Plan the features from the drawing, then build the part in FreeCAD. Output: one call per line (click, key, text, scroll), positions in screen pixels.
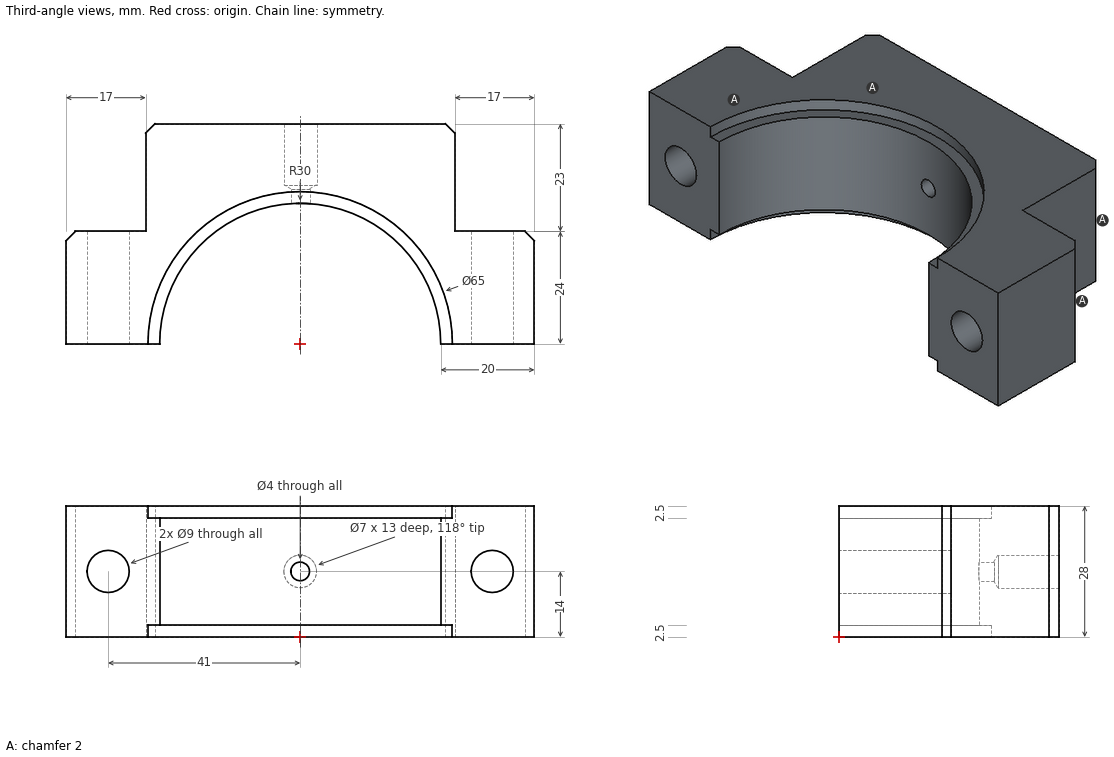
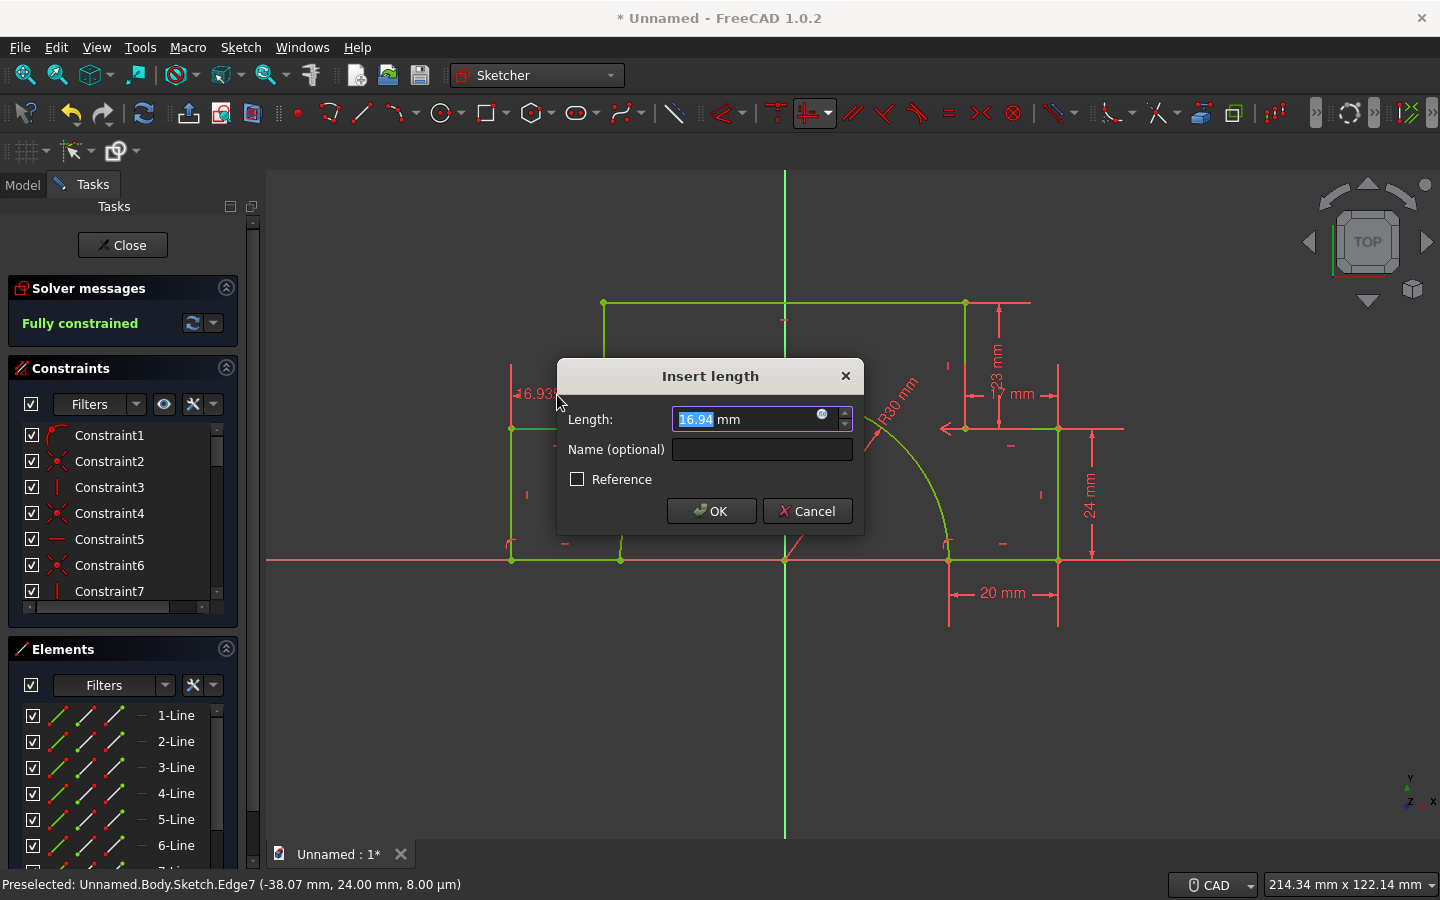
text(17)
key(Return)
key(Escape)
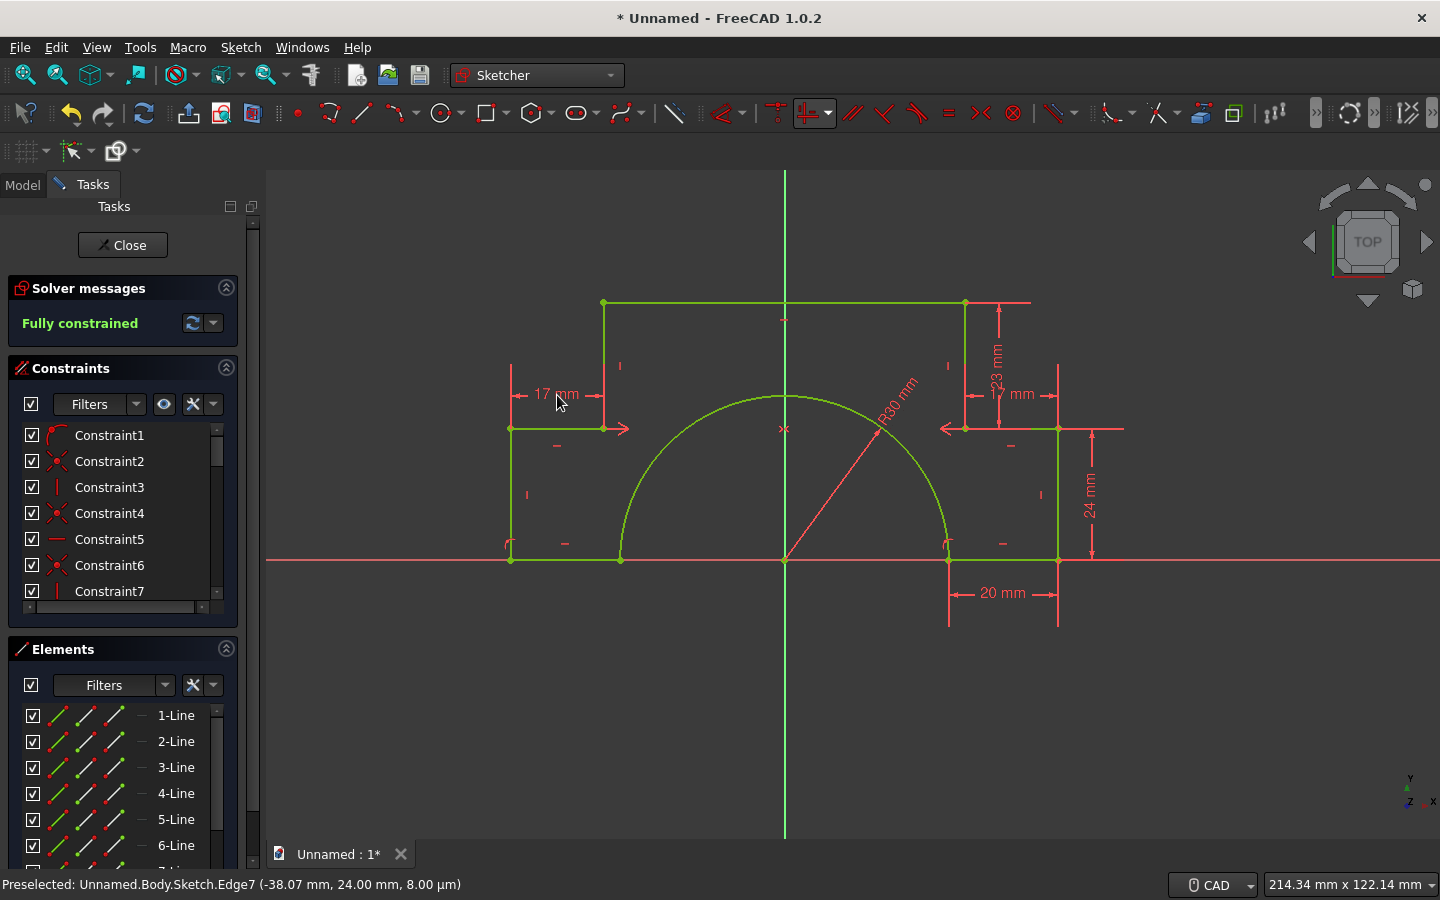
click(123, 245)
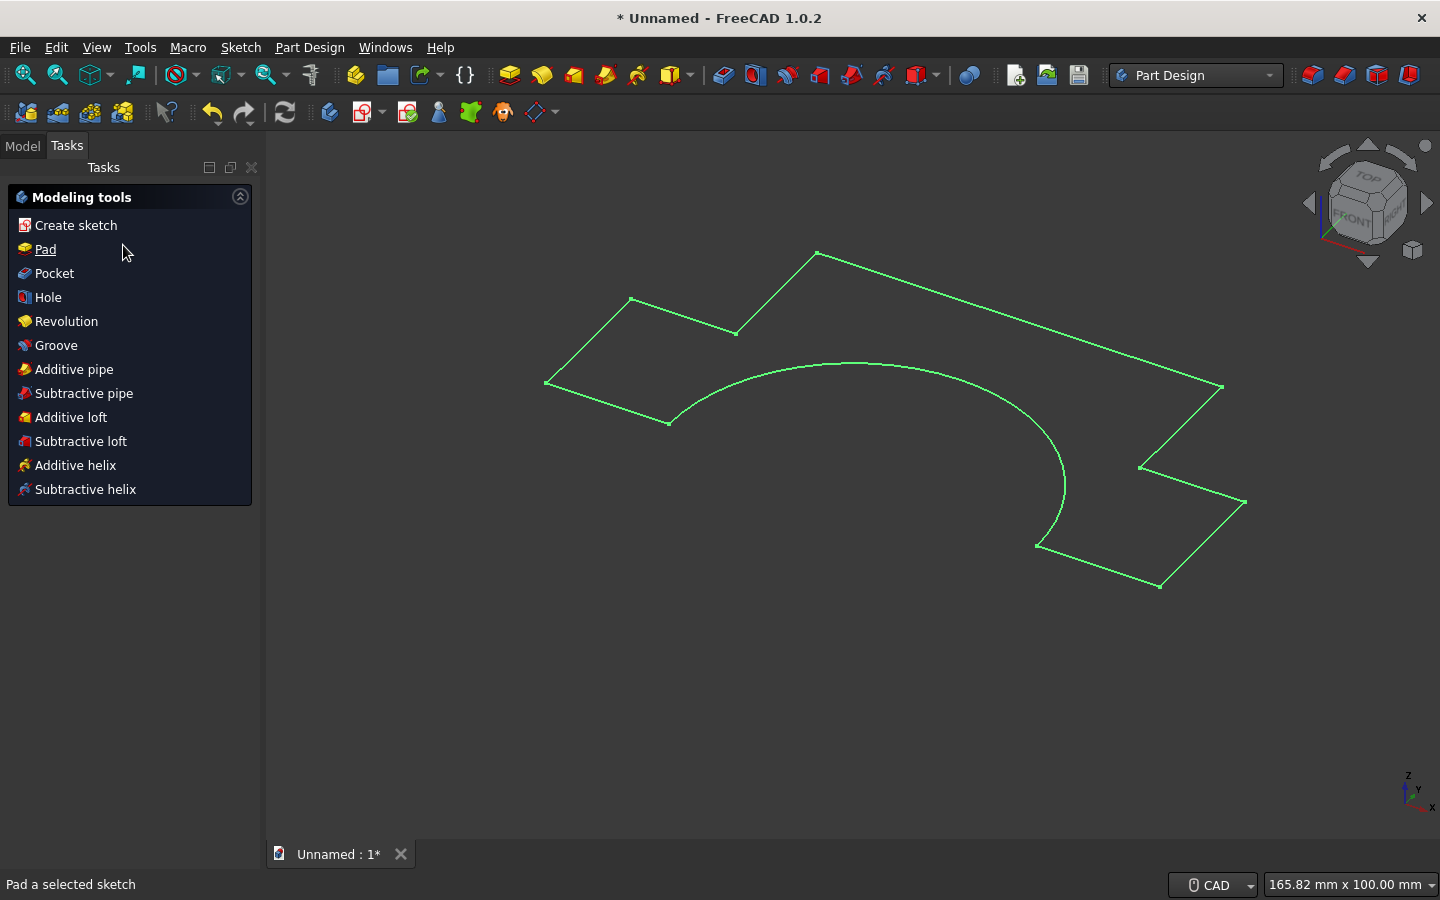
click(510, 76)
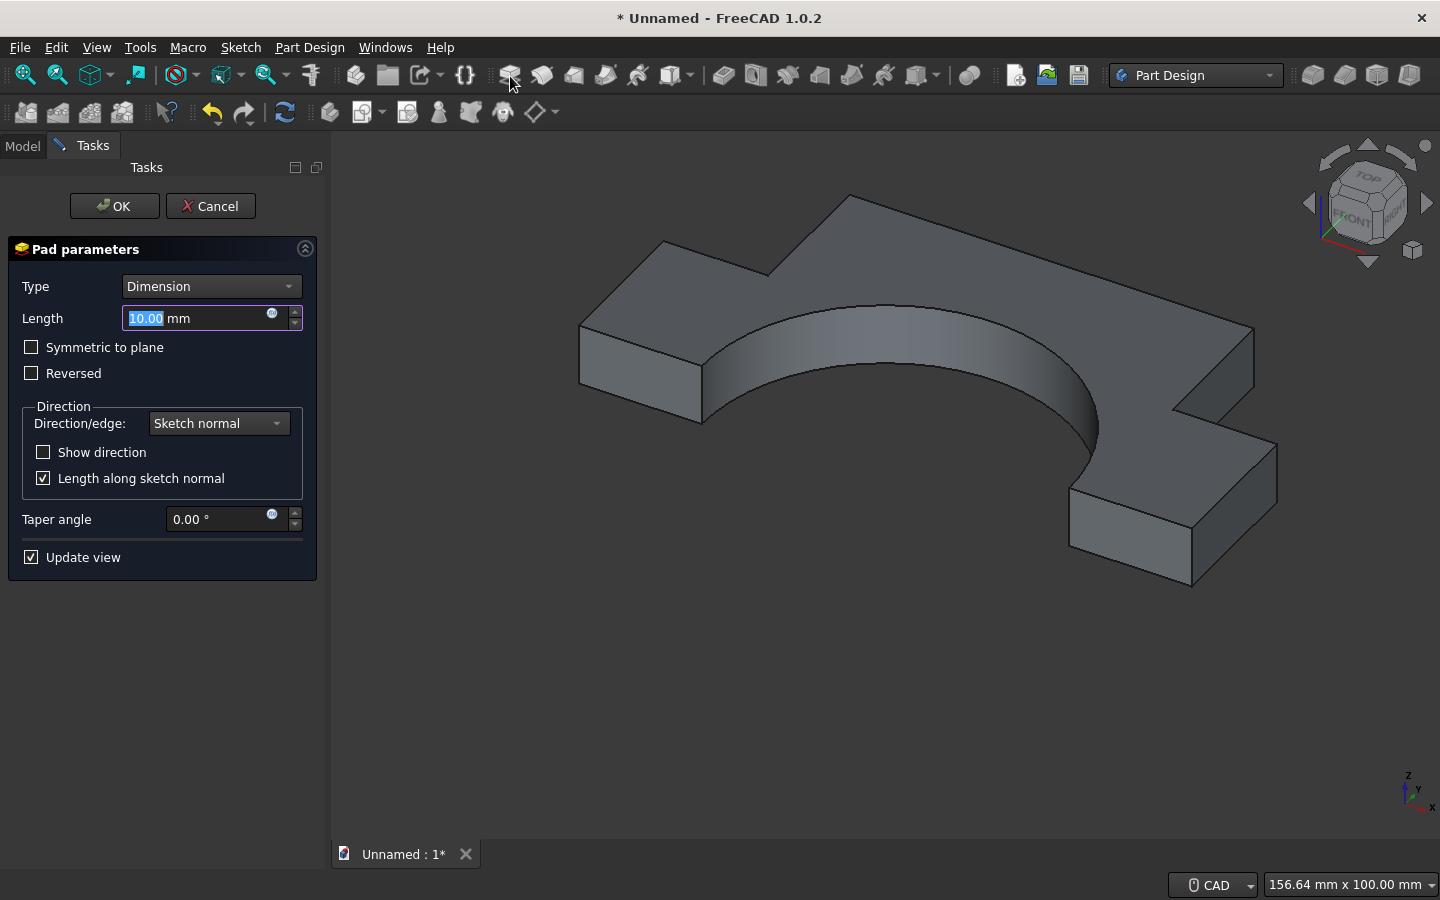
text(28)
key(Tab)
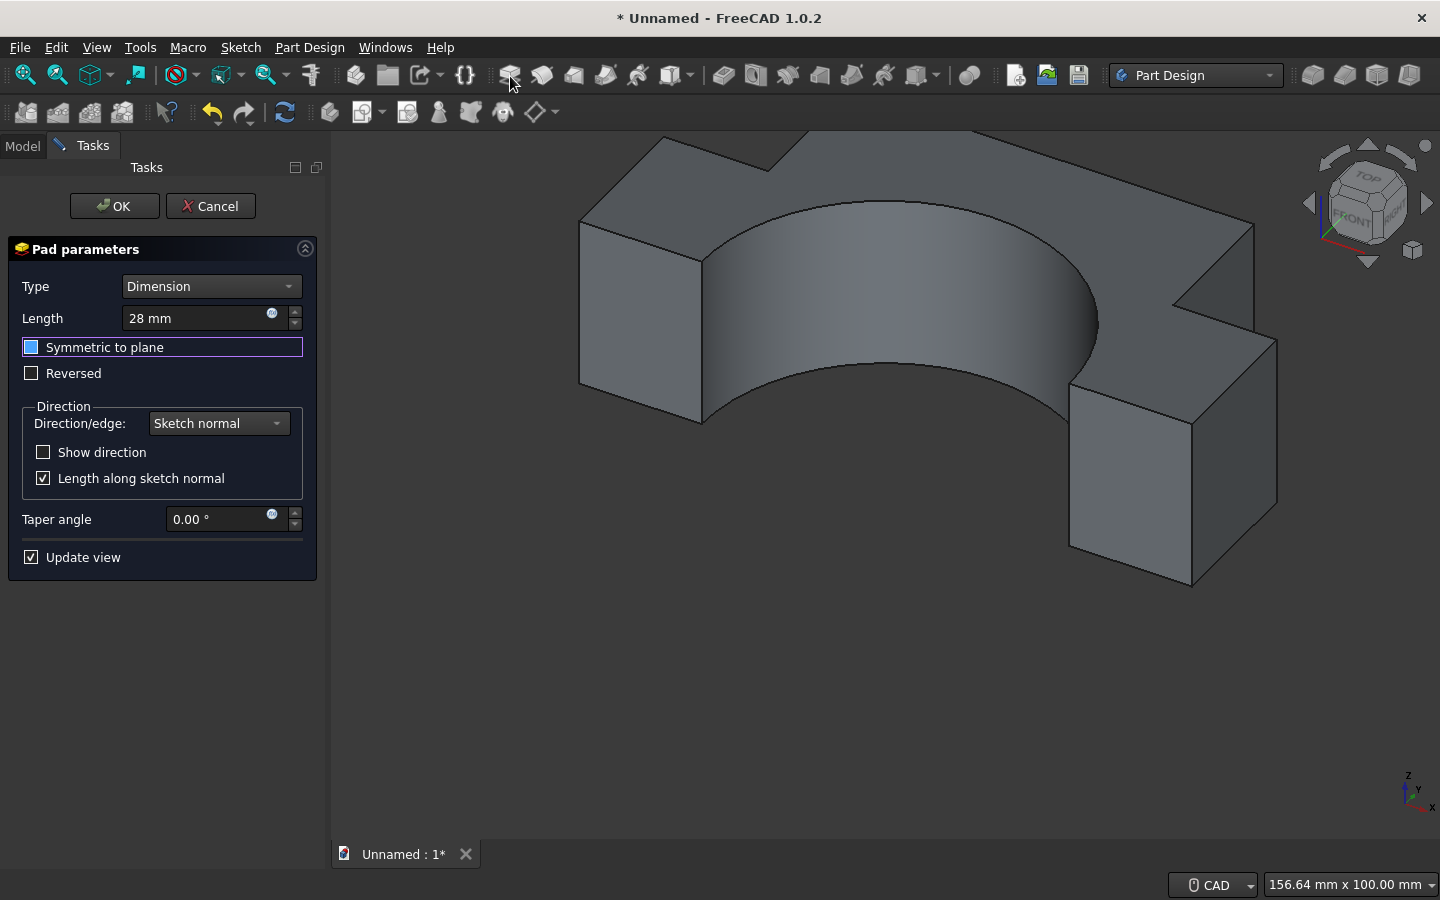
click(115, 206)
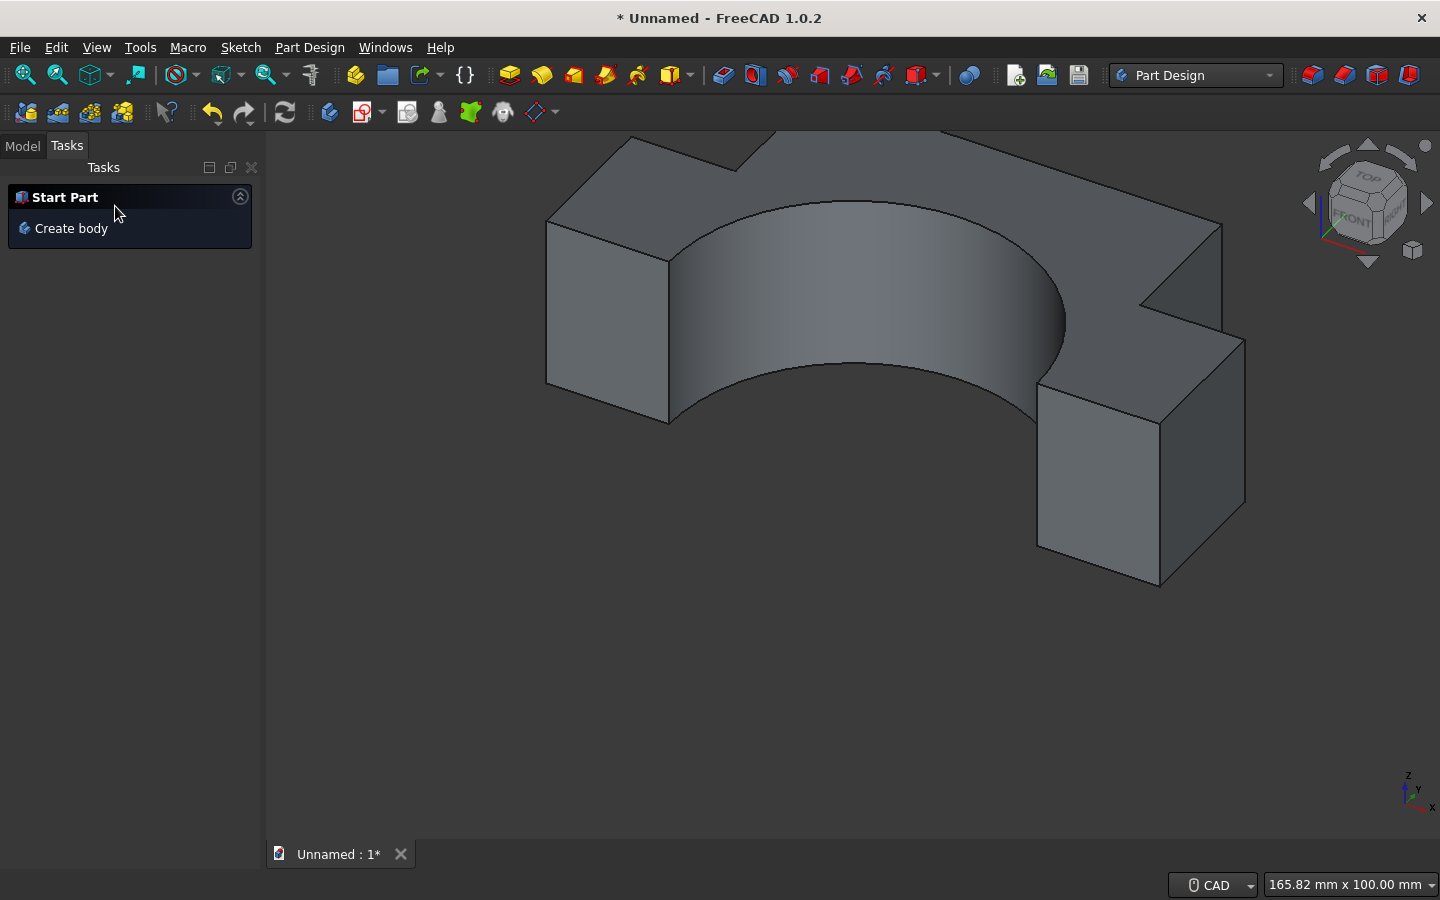
click(26, 76)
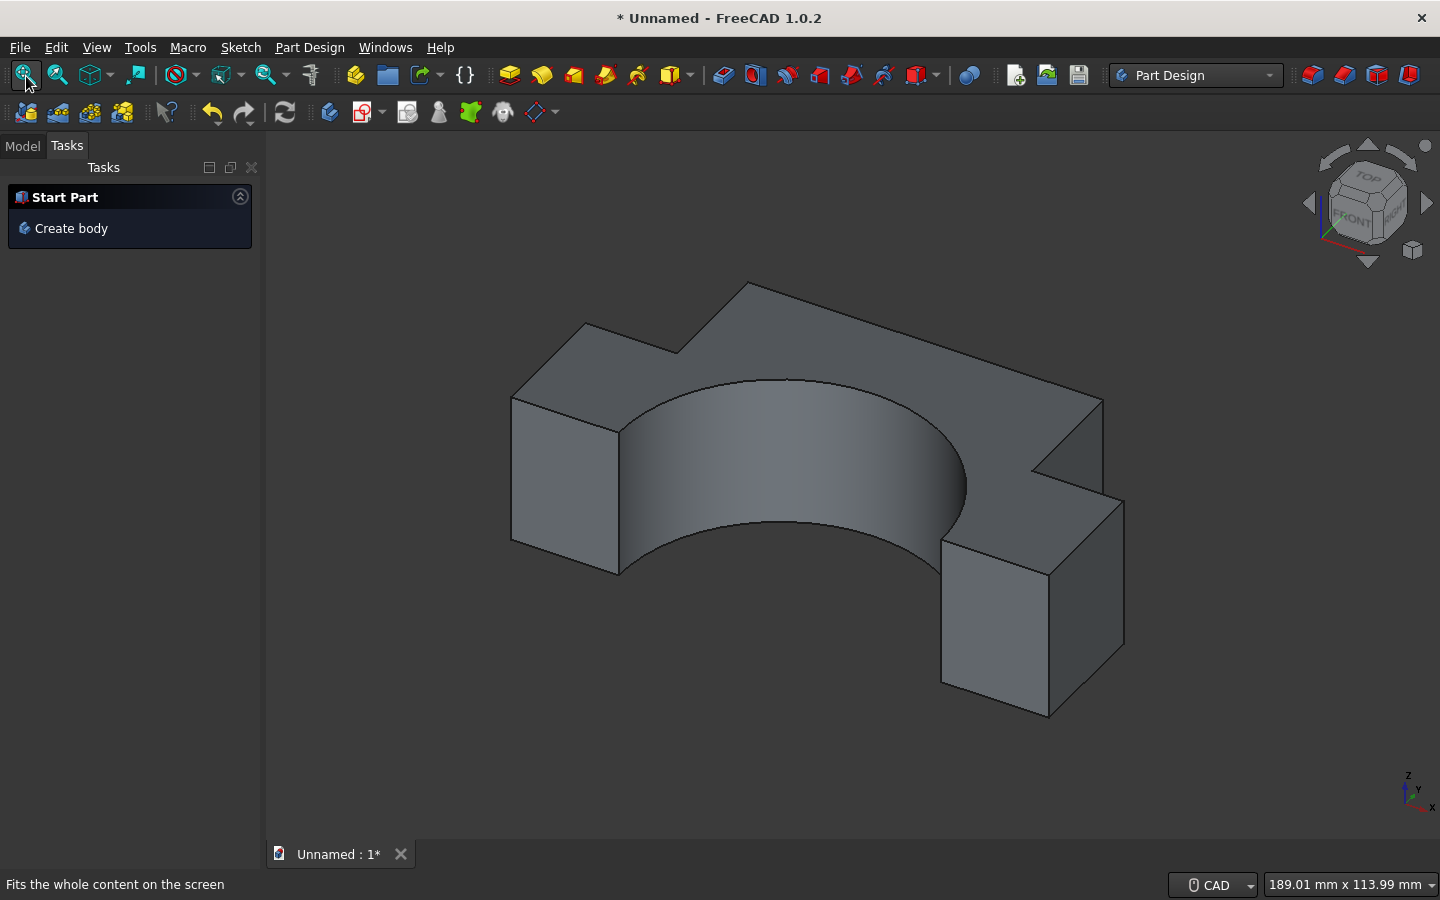
key(0)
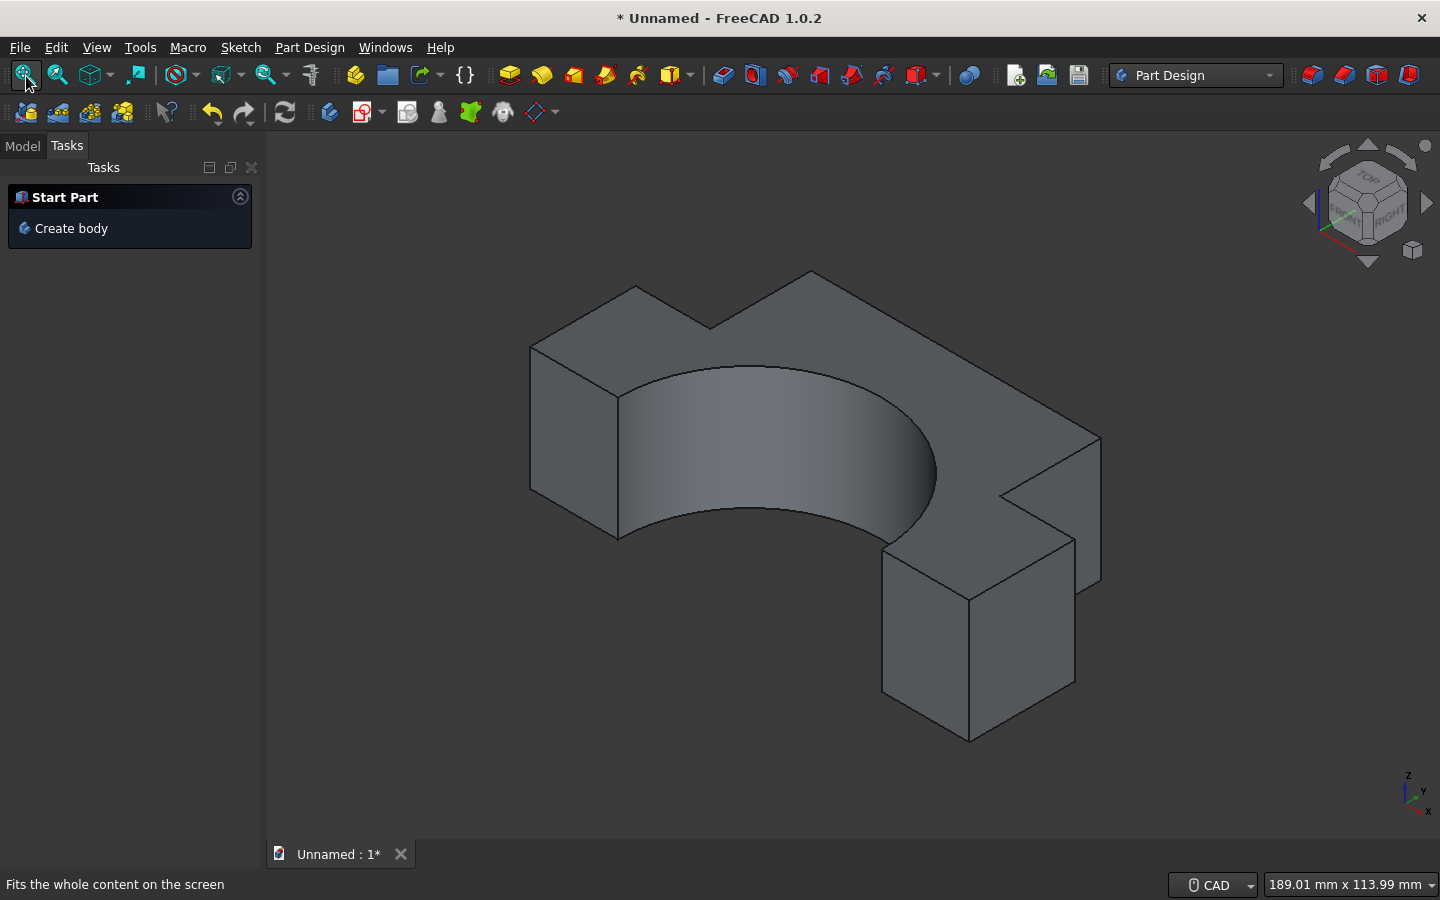
key(2)